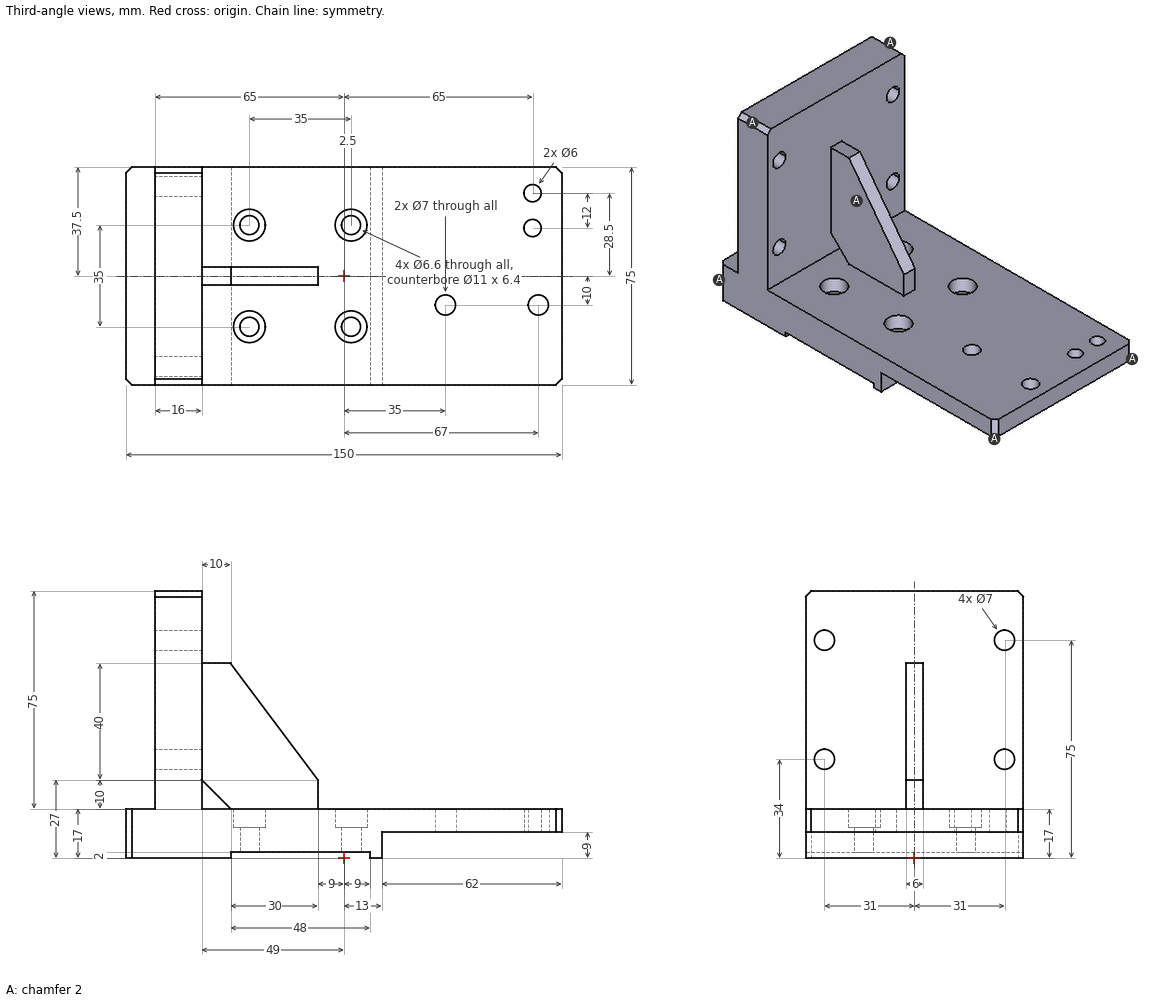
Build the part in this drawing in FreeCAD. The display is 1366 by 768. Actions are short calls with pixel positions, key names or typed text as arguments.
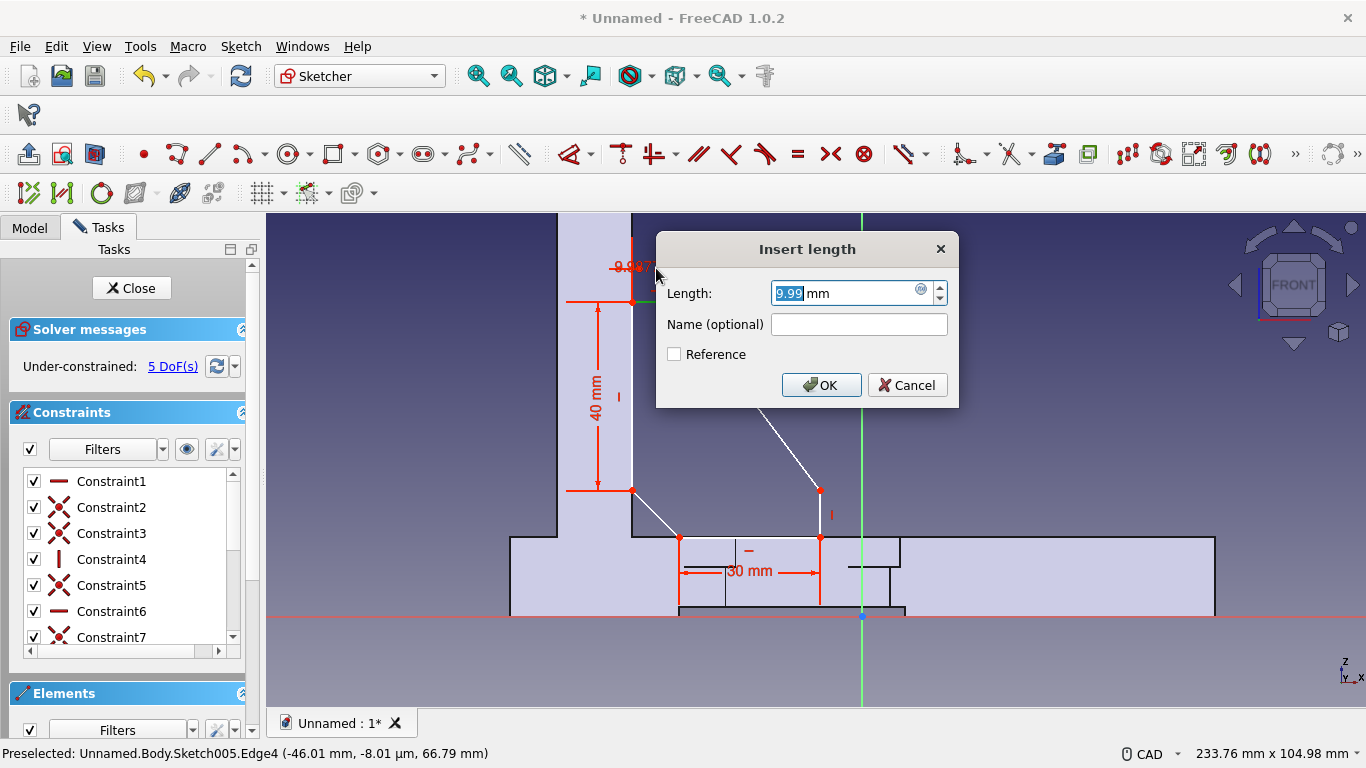
text(10)
key(Return)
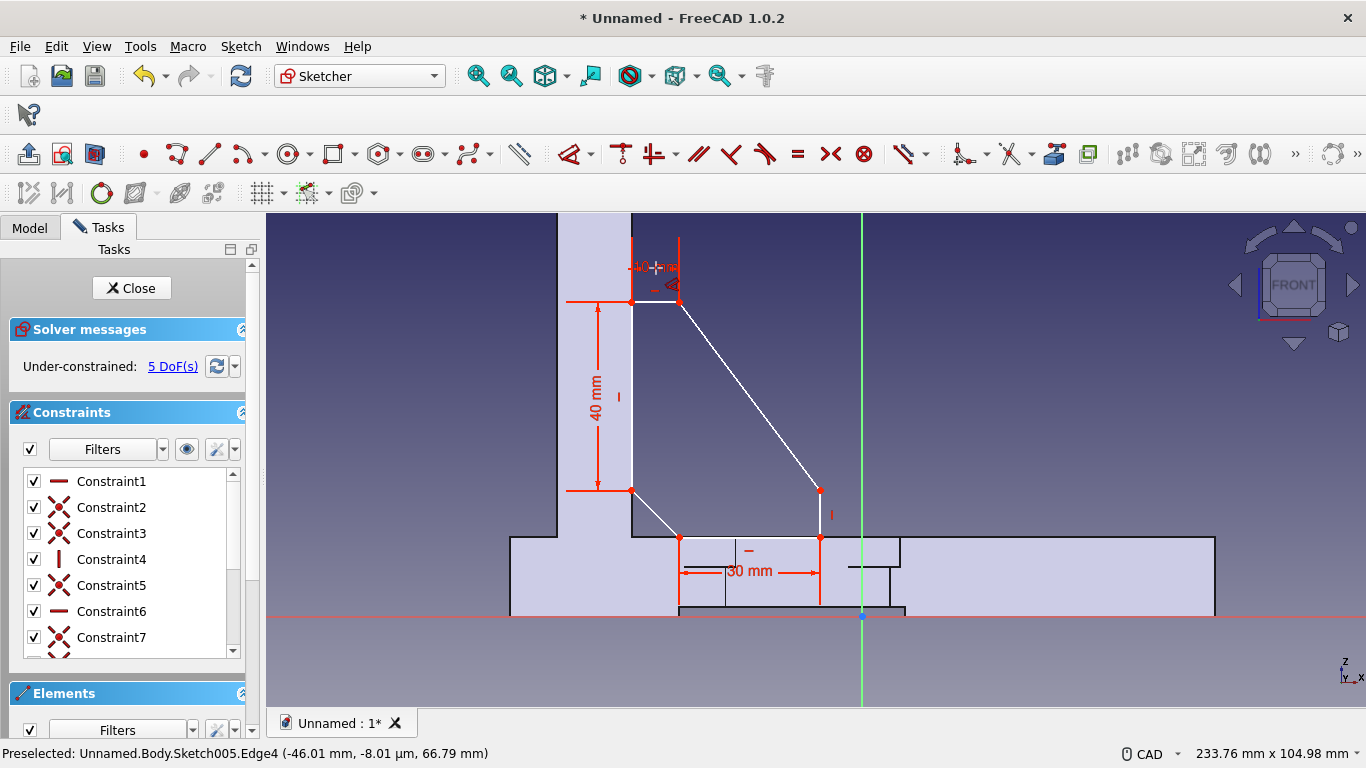
click(820, 505)
click(786, 514)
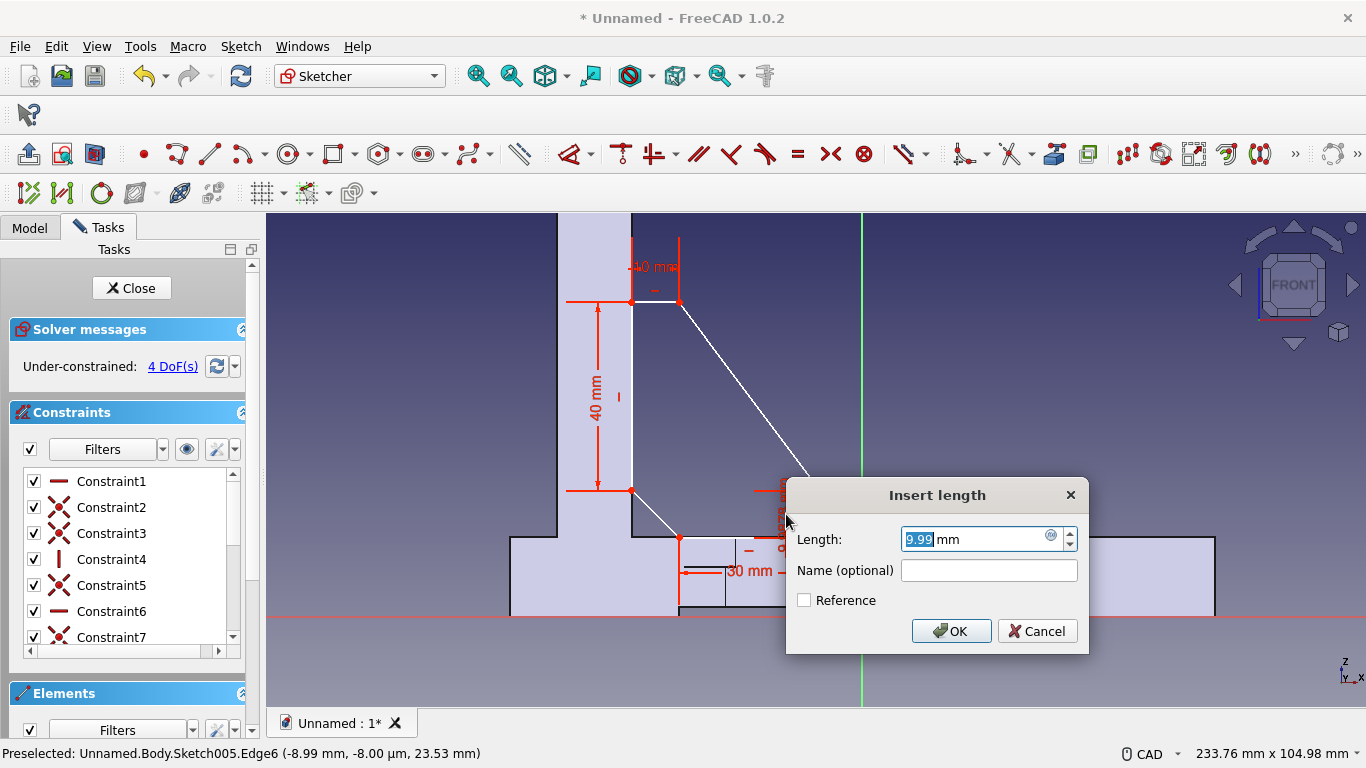
text(10)
key(Return)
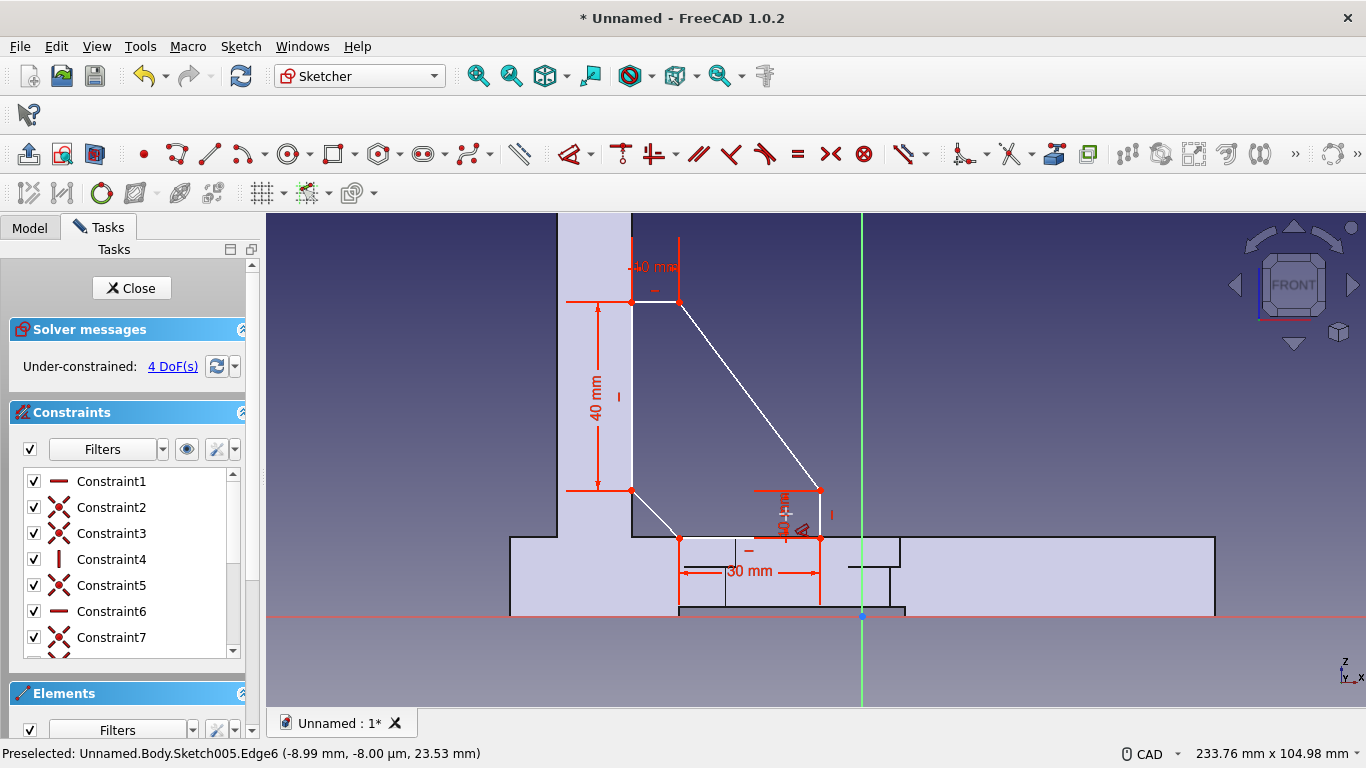
click(820, 538)
click(841, 651)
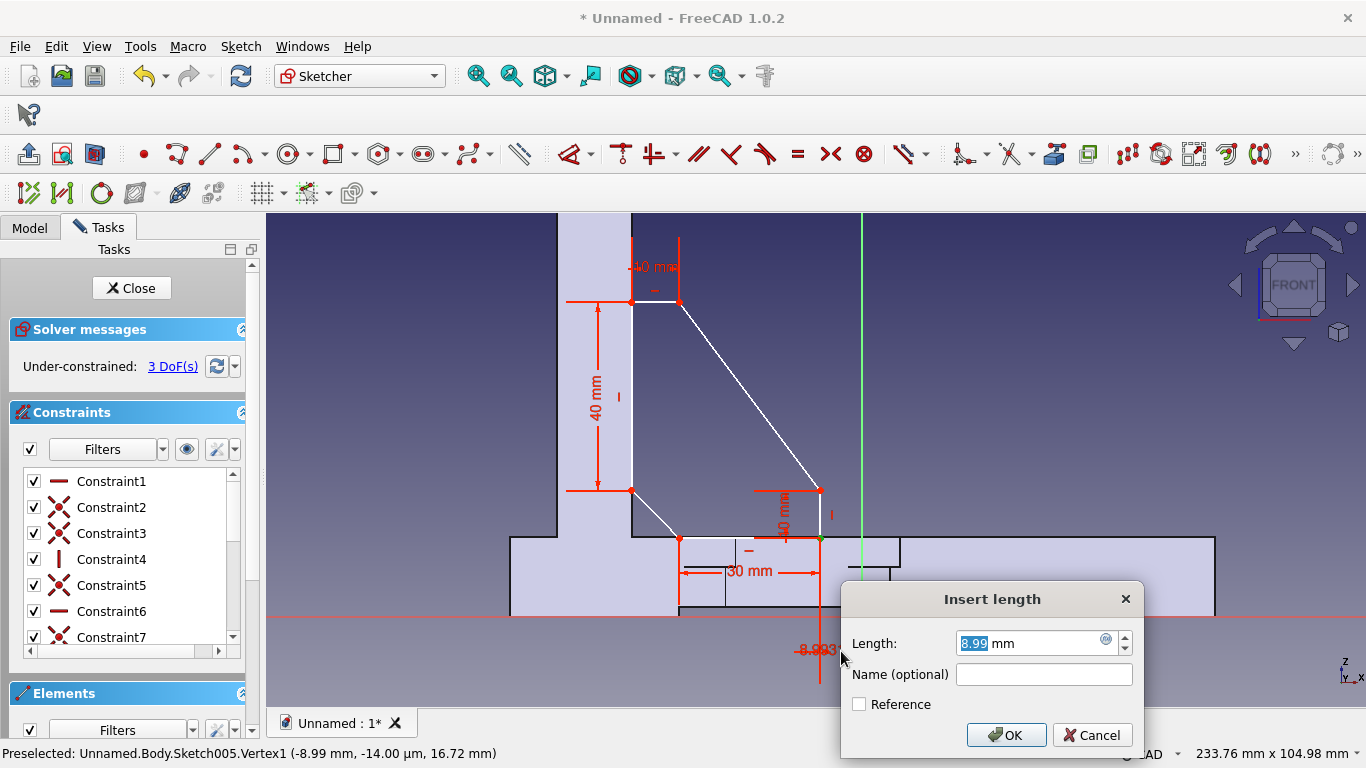
text(9)
key(Return)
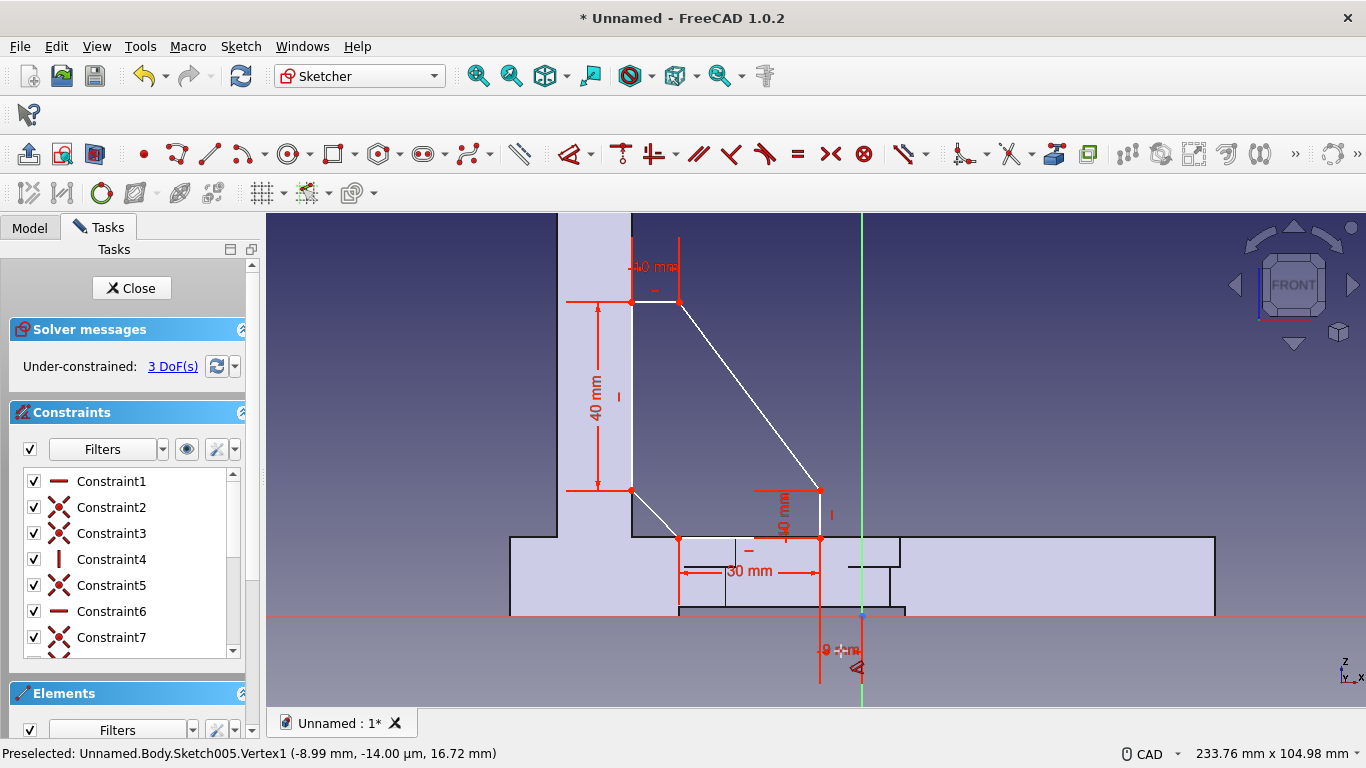
click(820, 538)
click(896, 577)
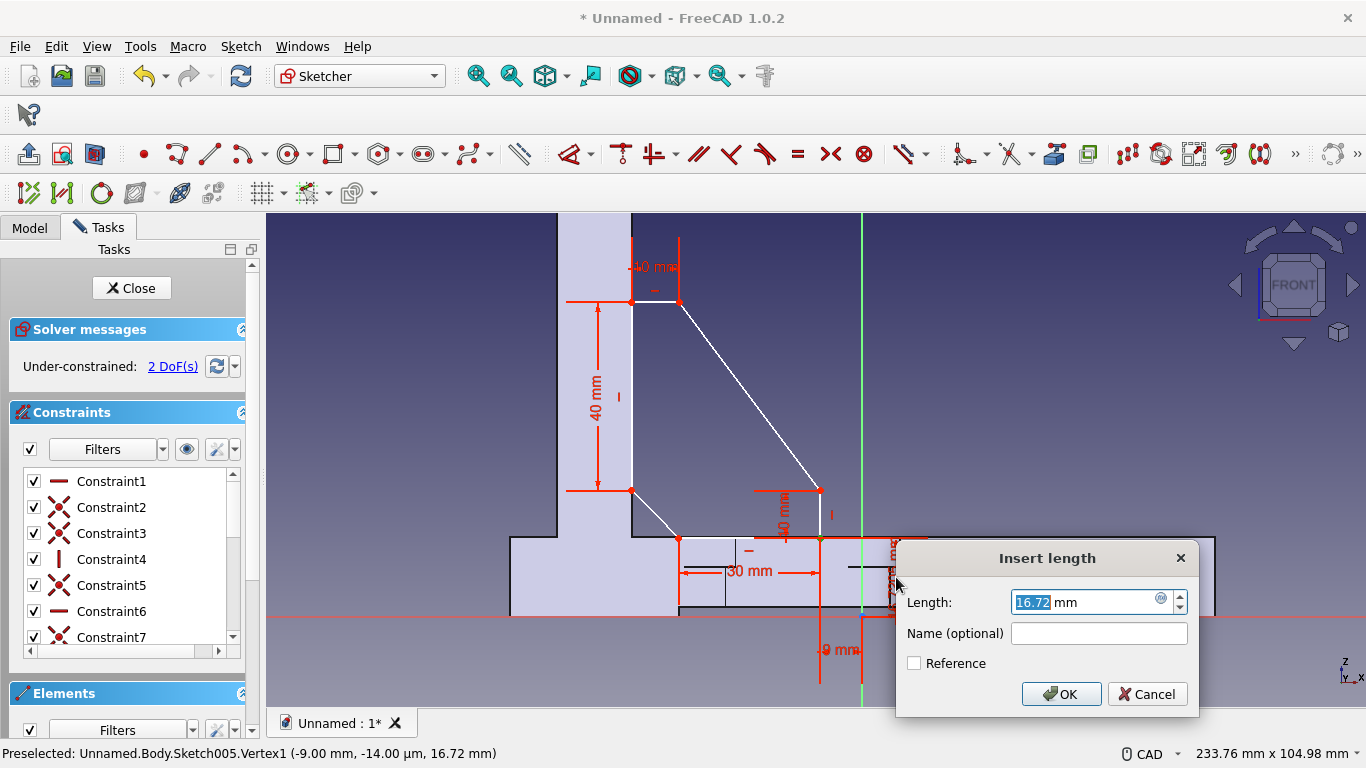
text(17)
key(Return)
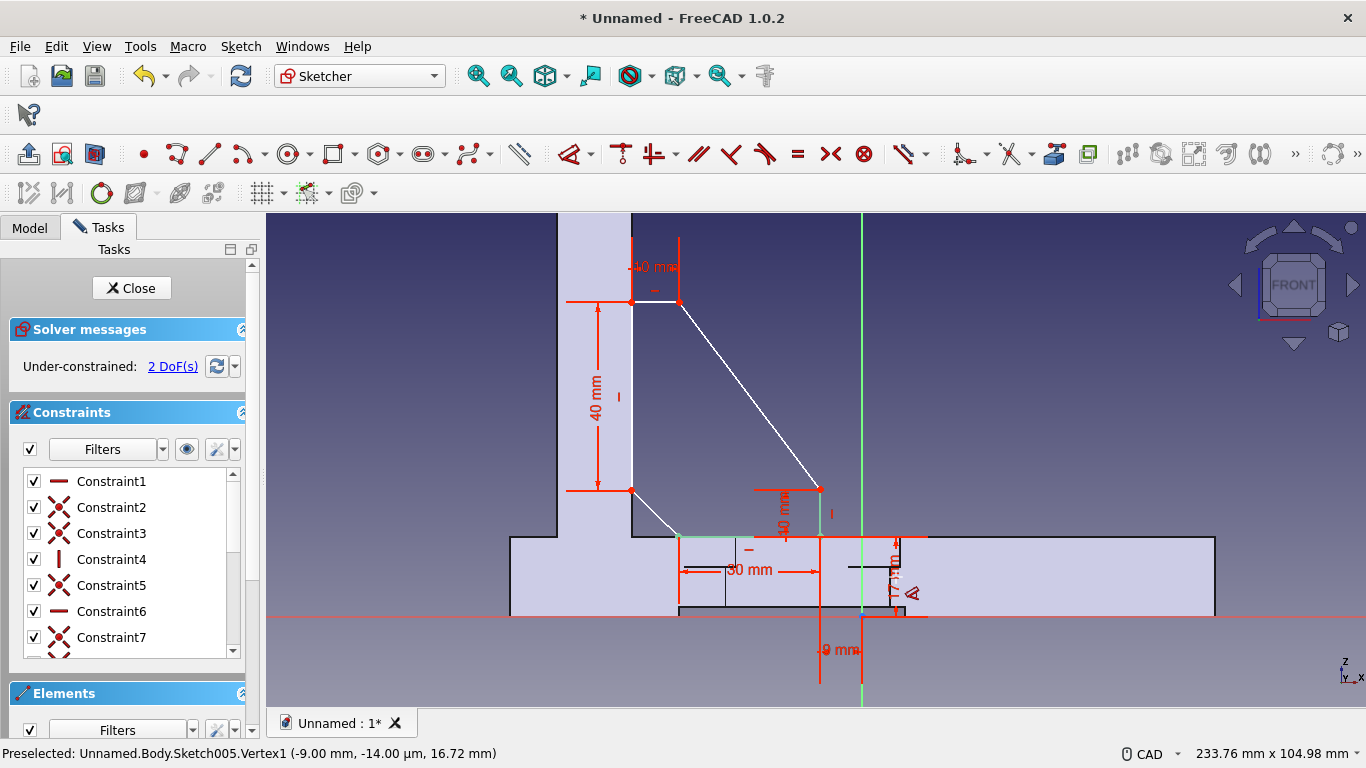
click(632, 491)
click(747, 651)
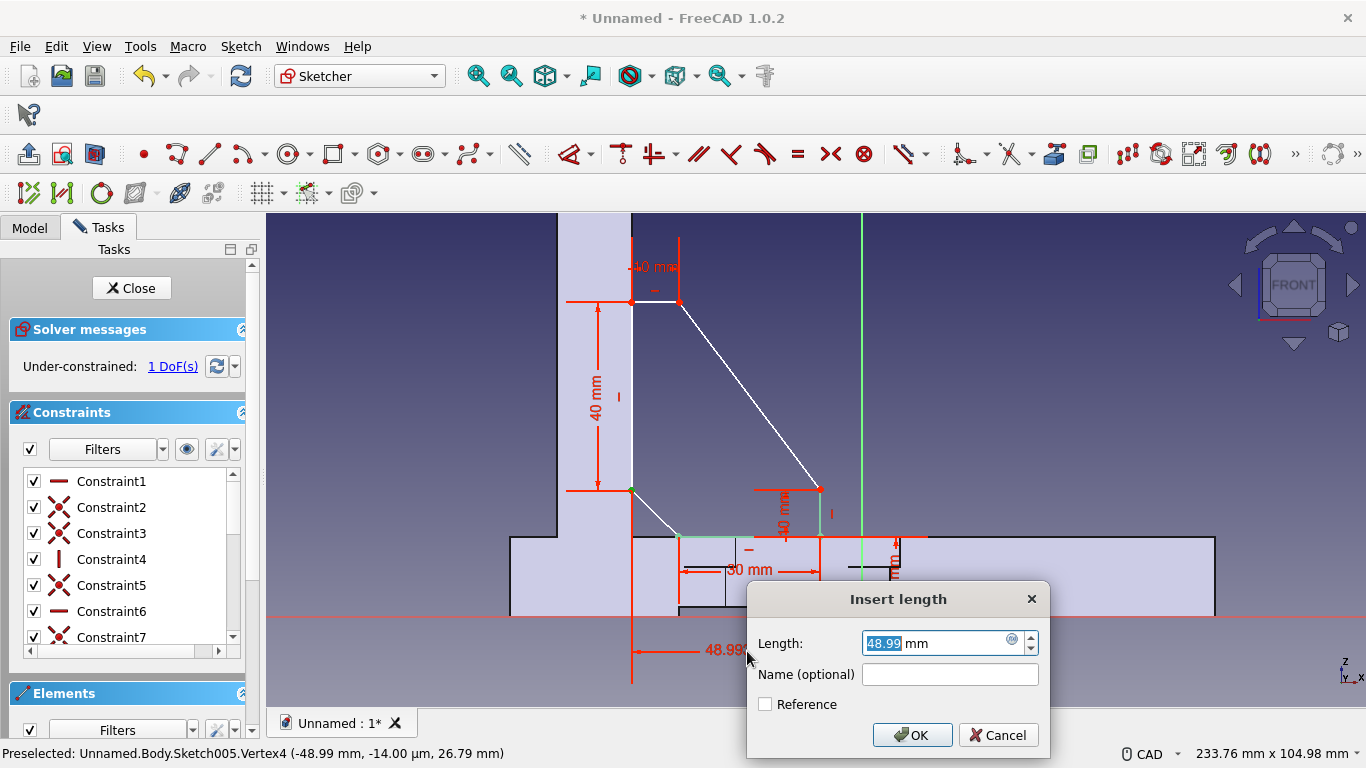
text(49)
key(Return)